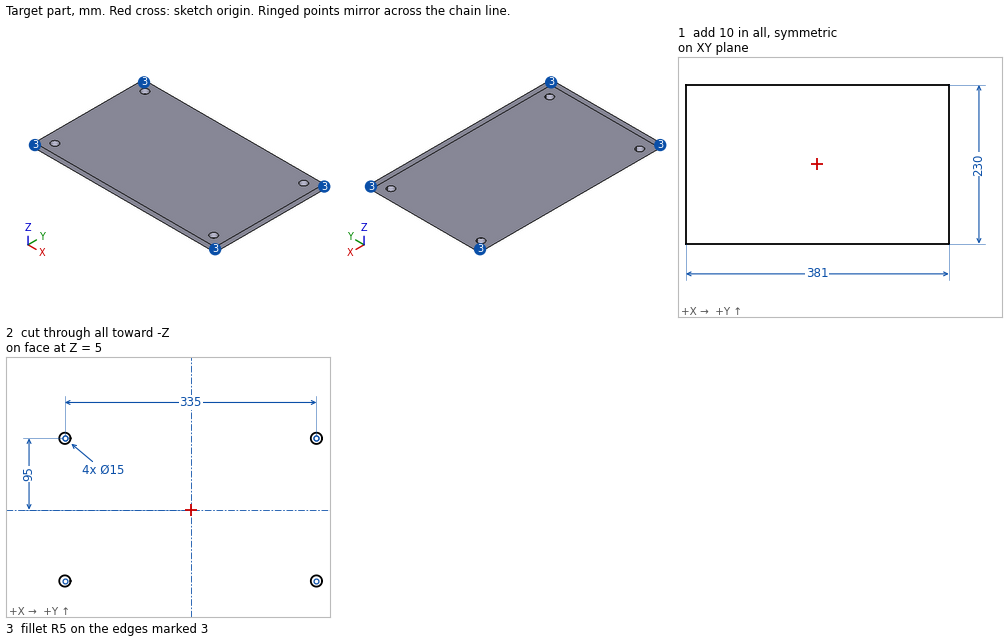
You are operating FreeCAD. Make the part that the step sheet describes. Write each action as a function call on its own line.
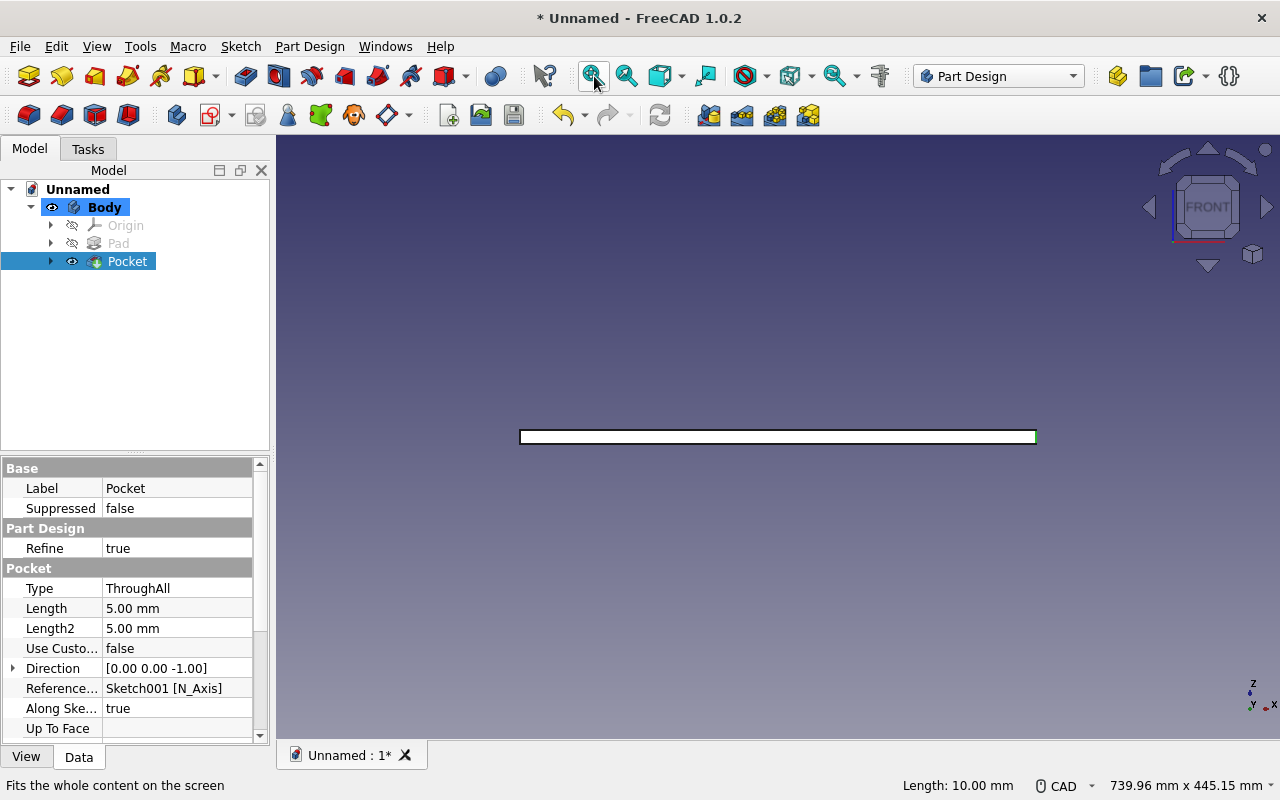
click(520, 436, ctrl)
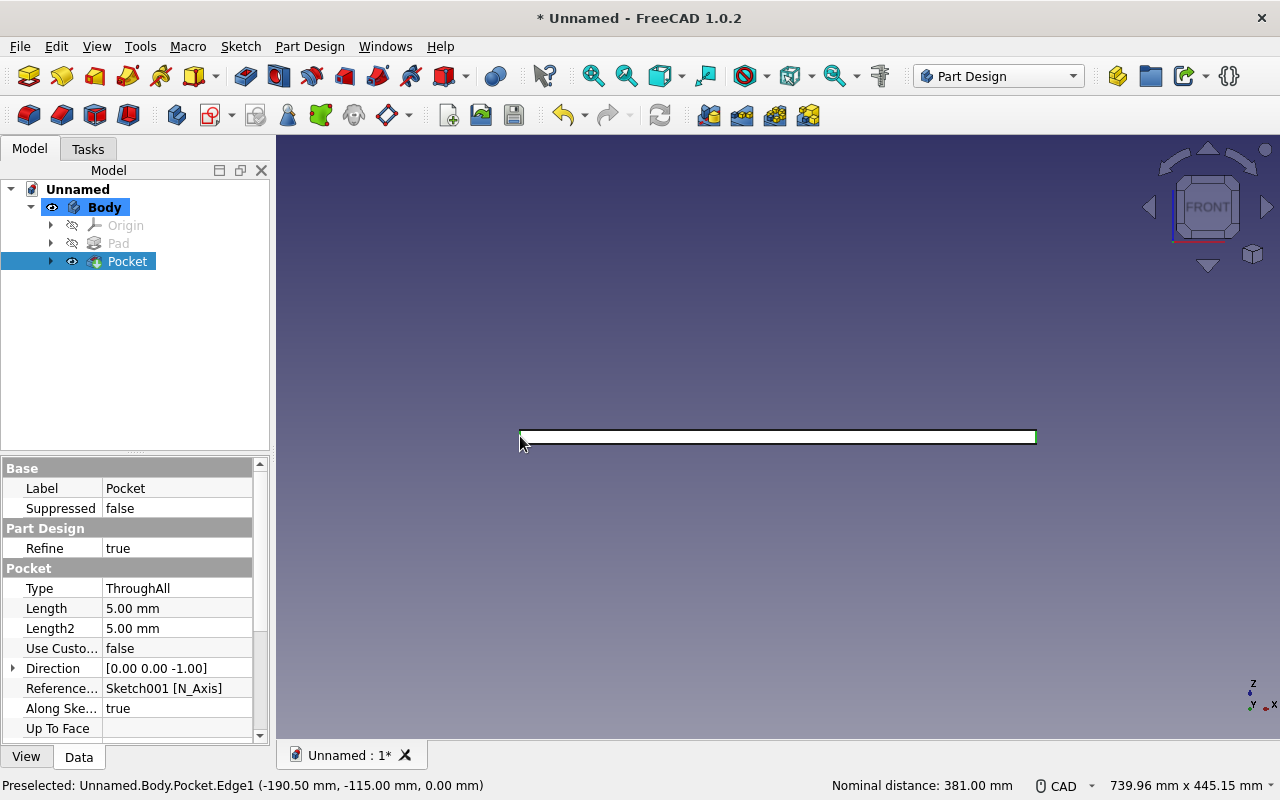
scroll(520, 436, up, 6)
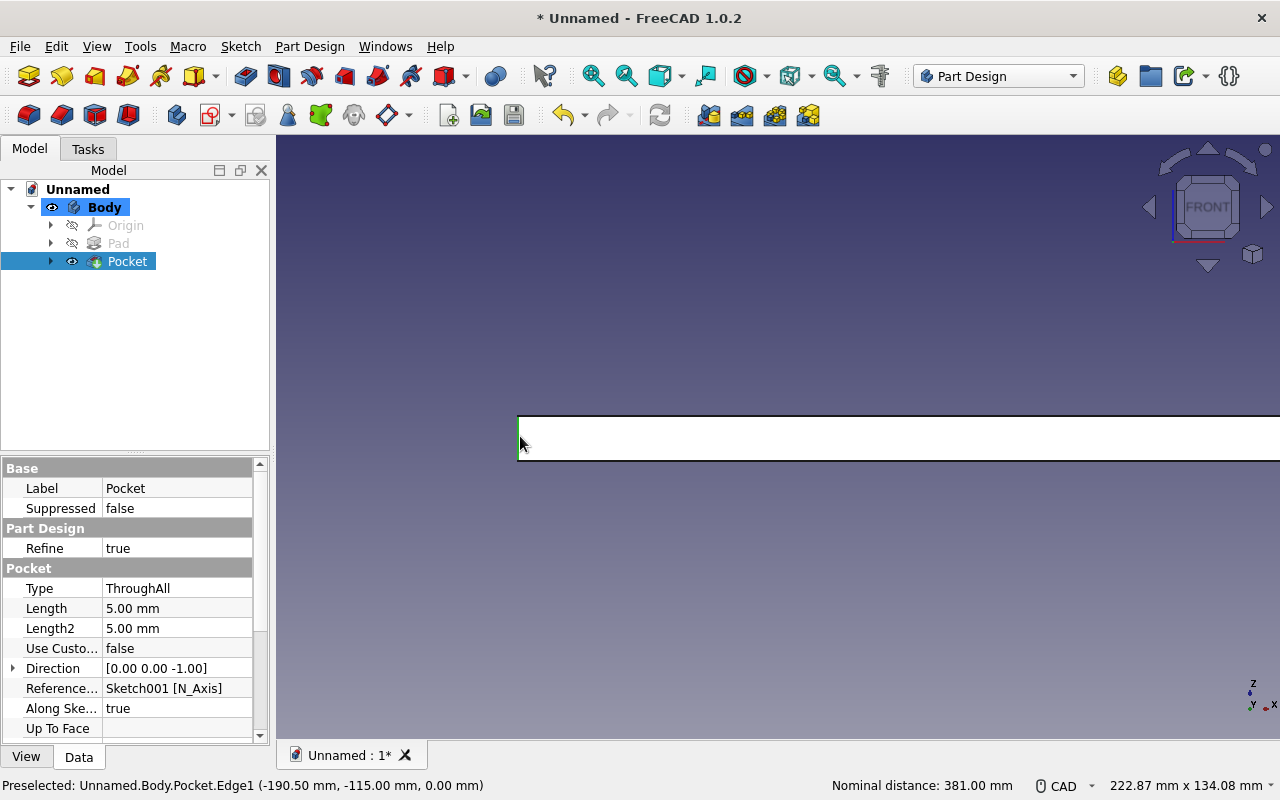
click(594, 76)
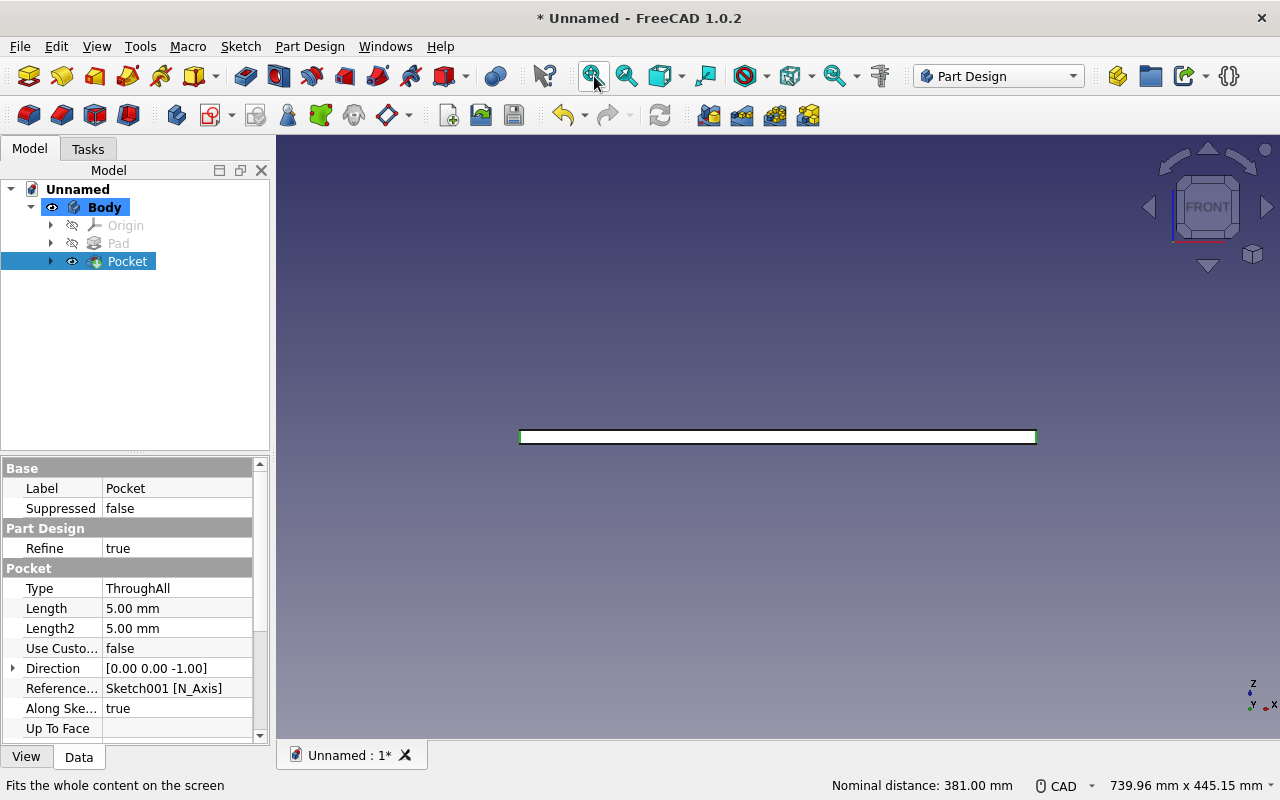
key(3)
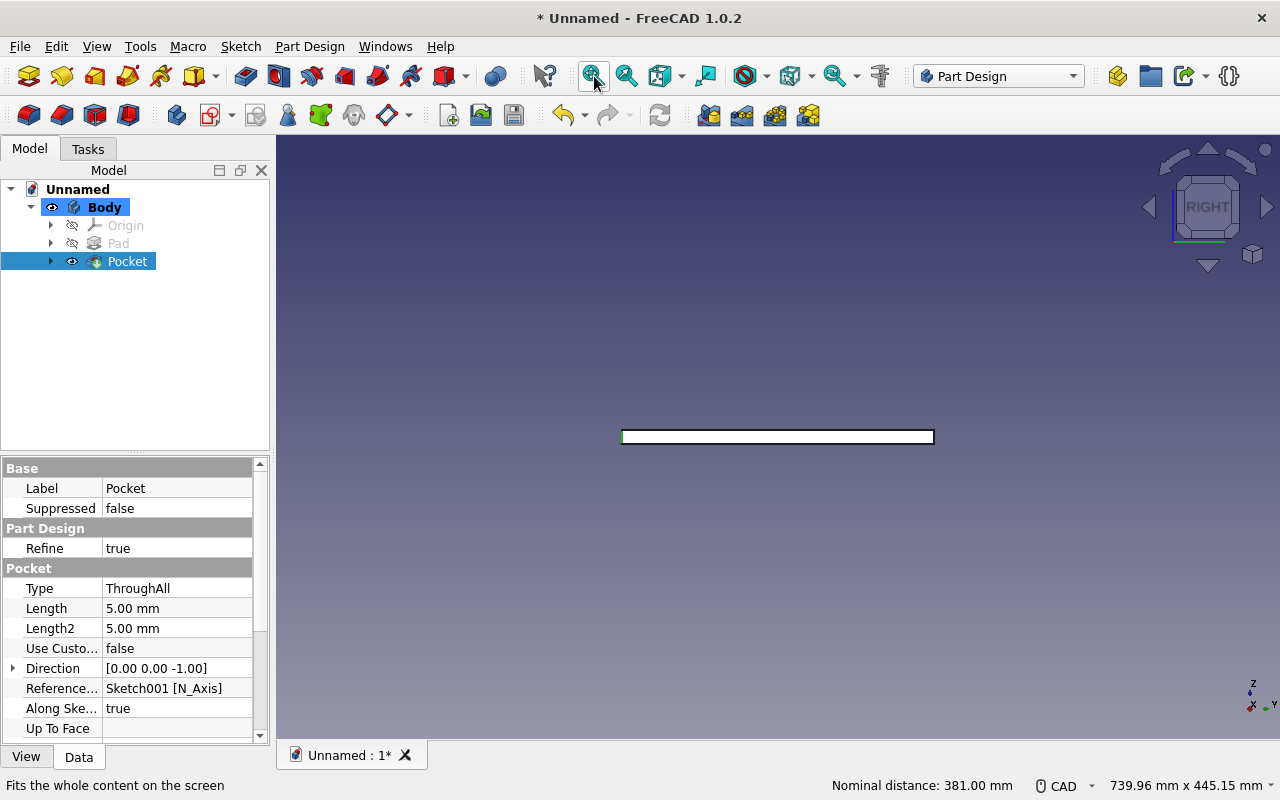
click(594, 76)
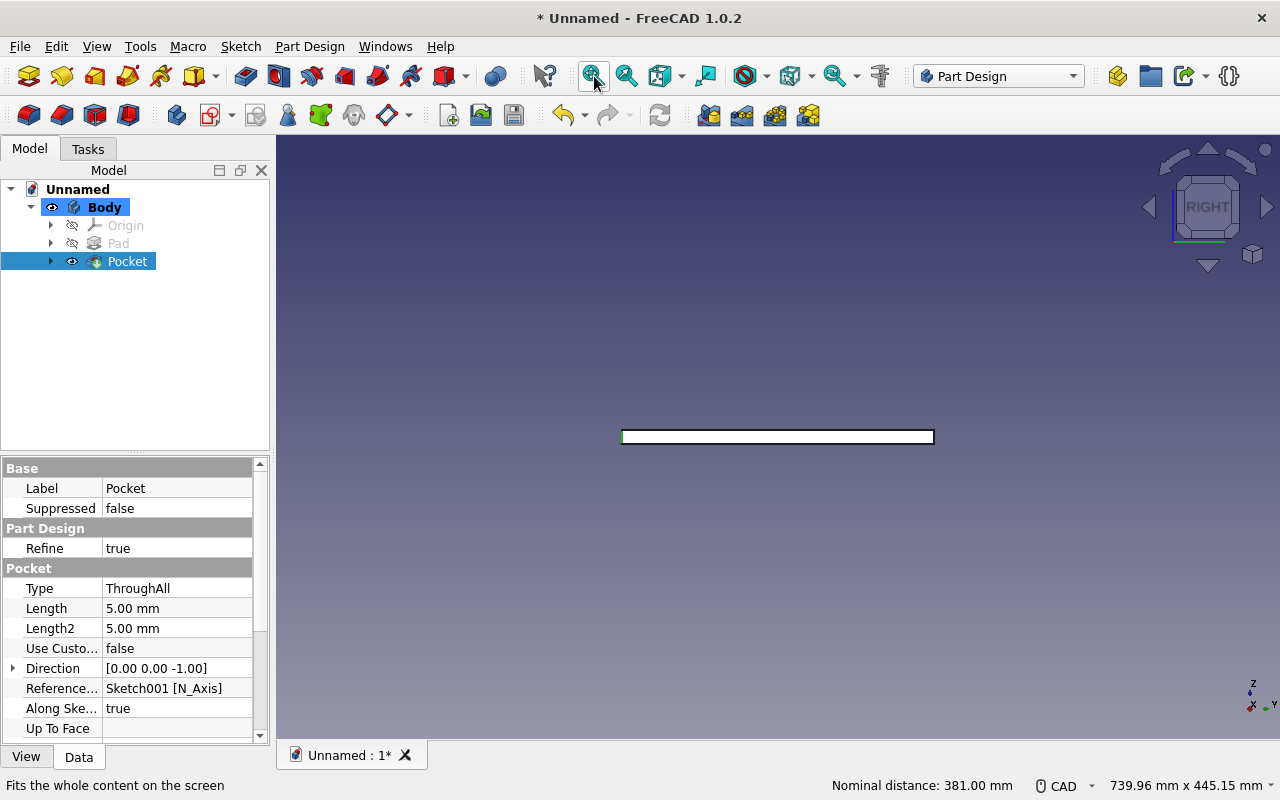
click(934, 436, ctrl)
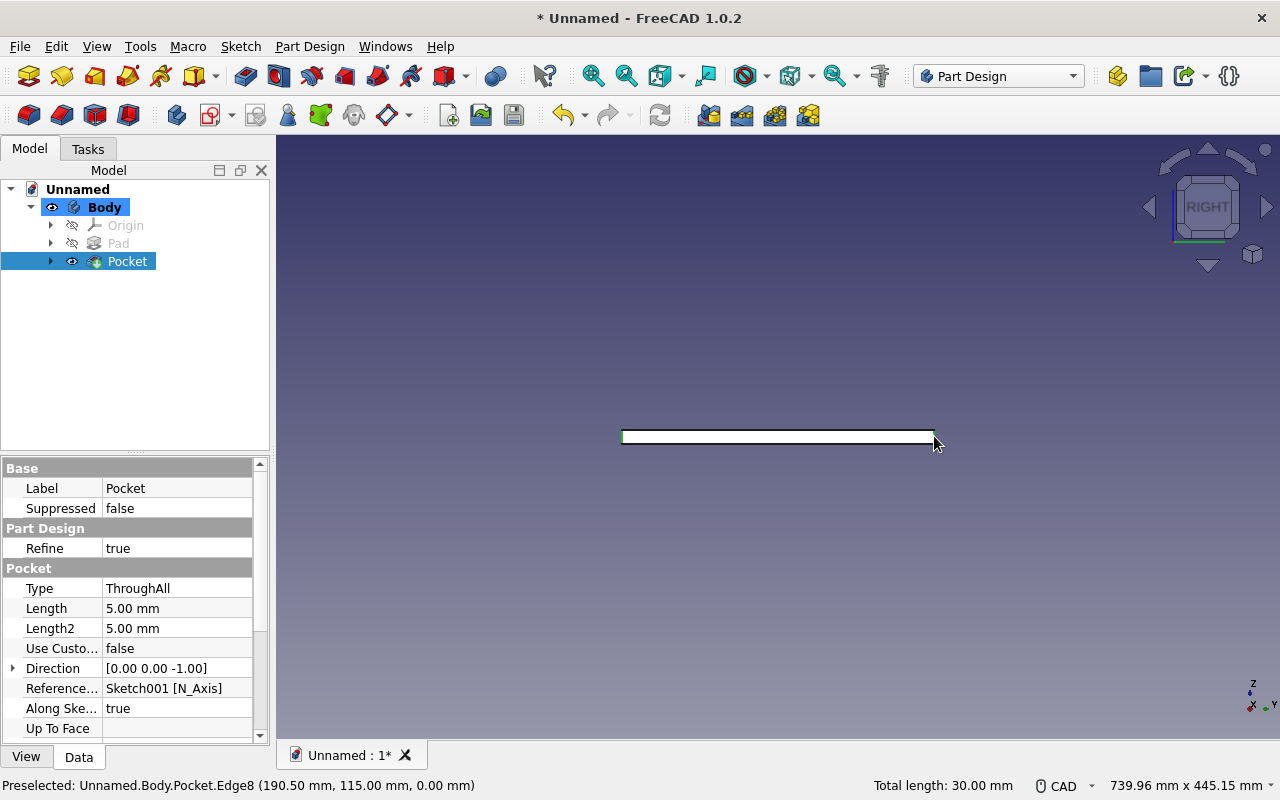
scroll(934, 436, up, 6)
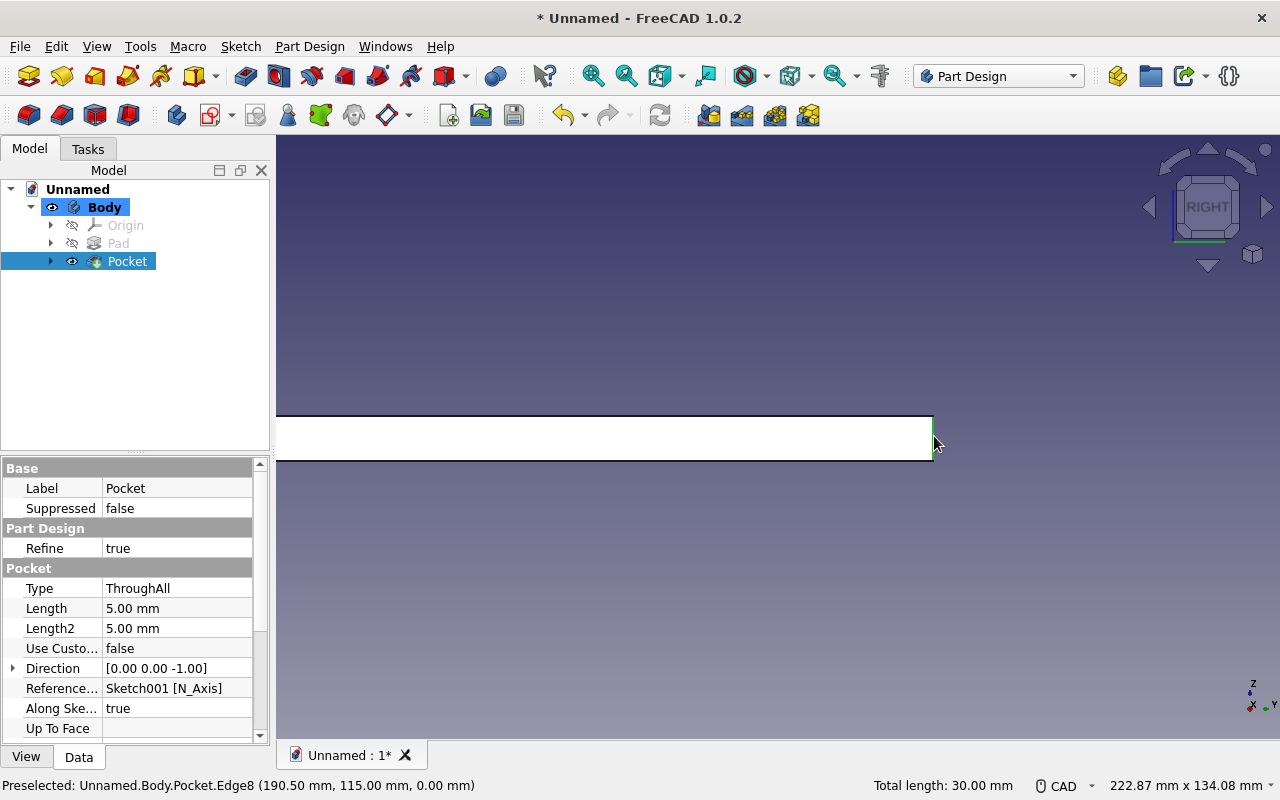
click(594, 76)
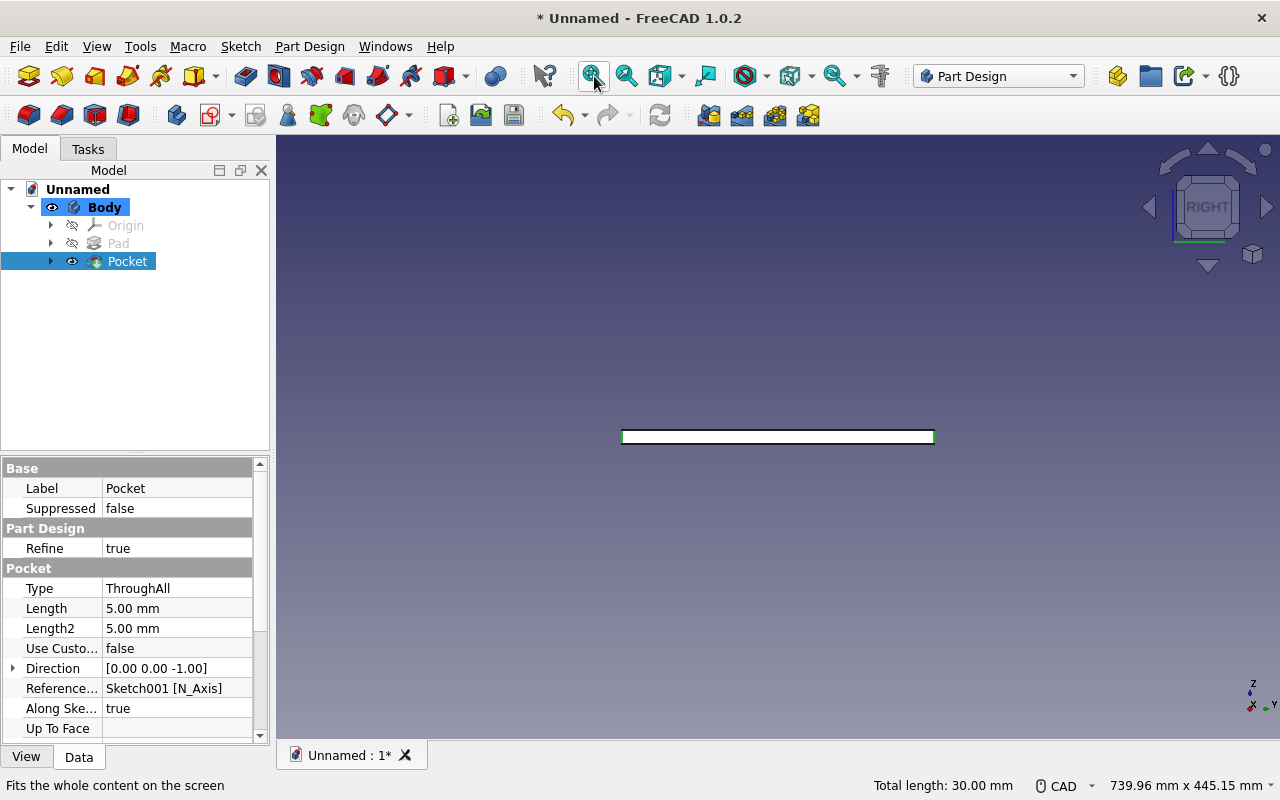
key(5)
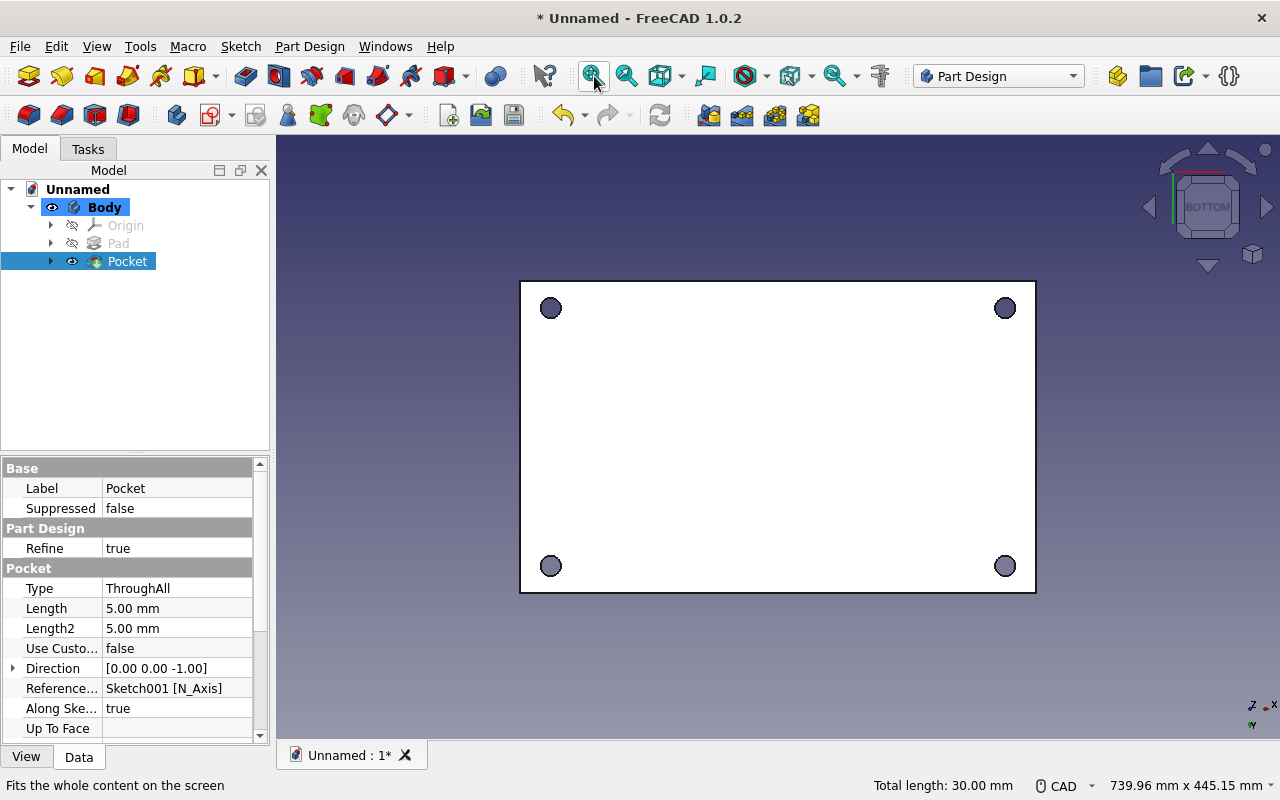
scroll(520, 592, up, 6)